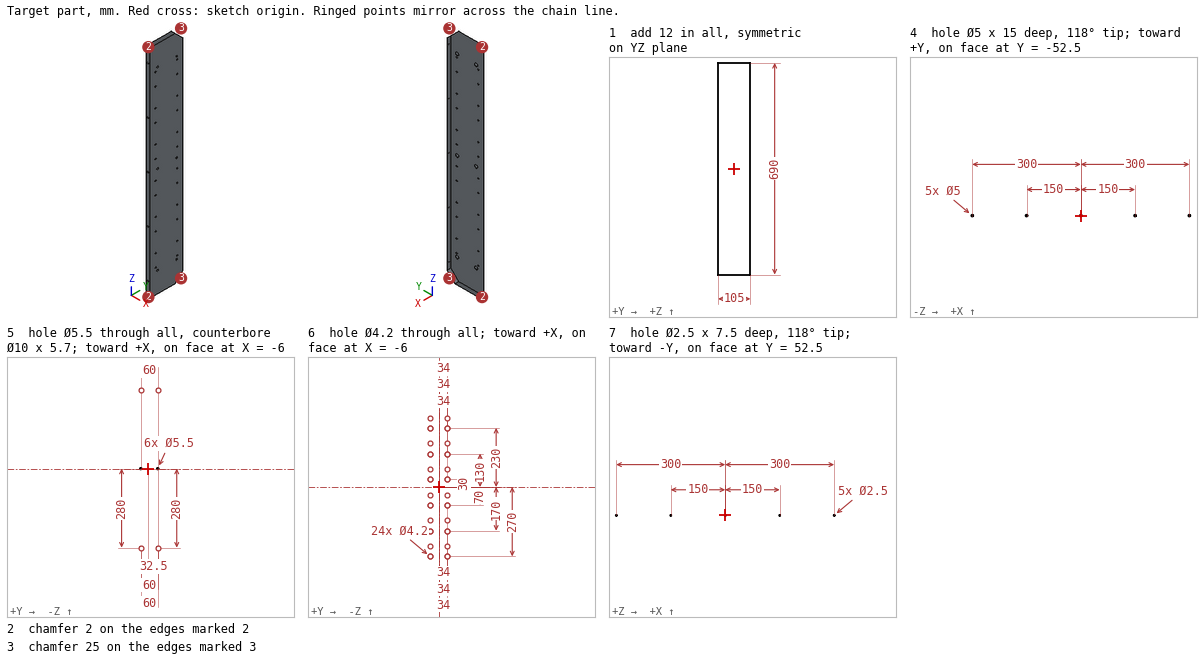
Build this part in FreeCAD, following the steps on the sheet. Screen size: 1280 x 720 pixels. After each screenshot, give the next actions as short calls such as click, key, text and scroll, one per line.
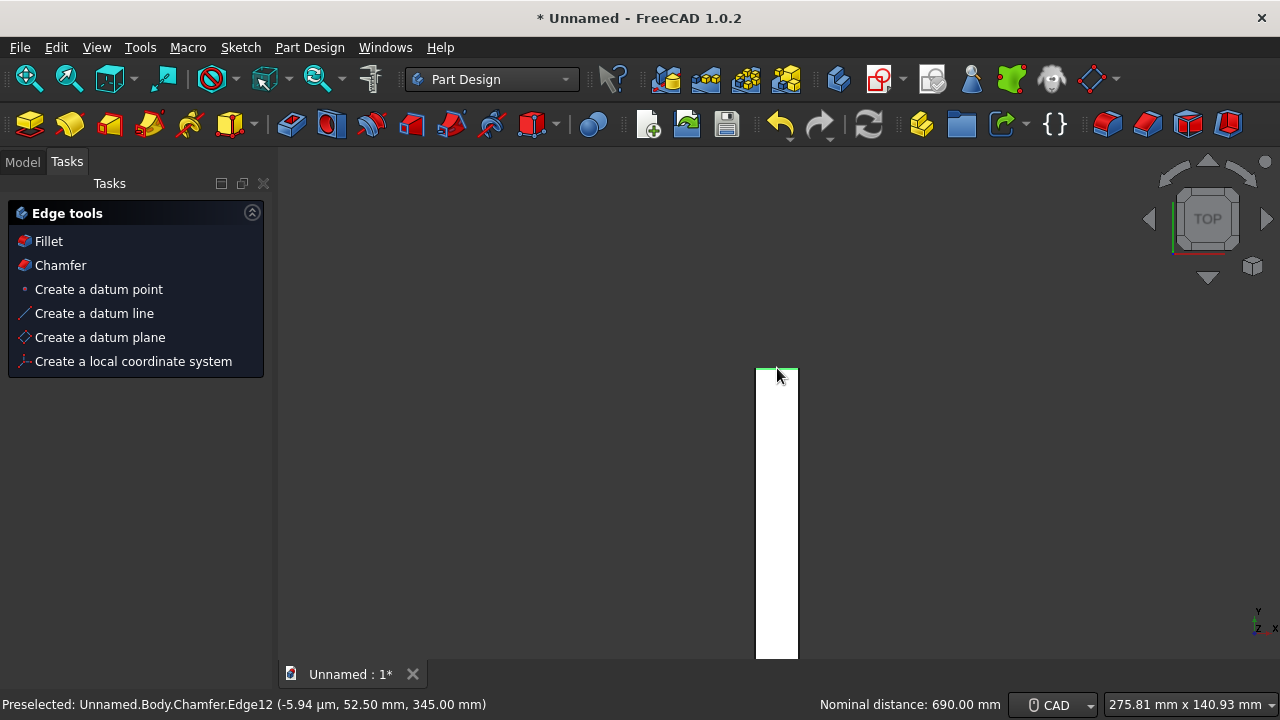
click(1148, 124)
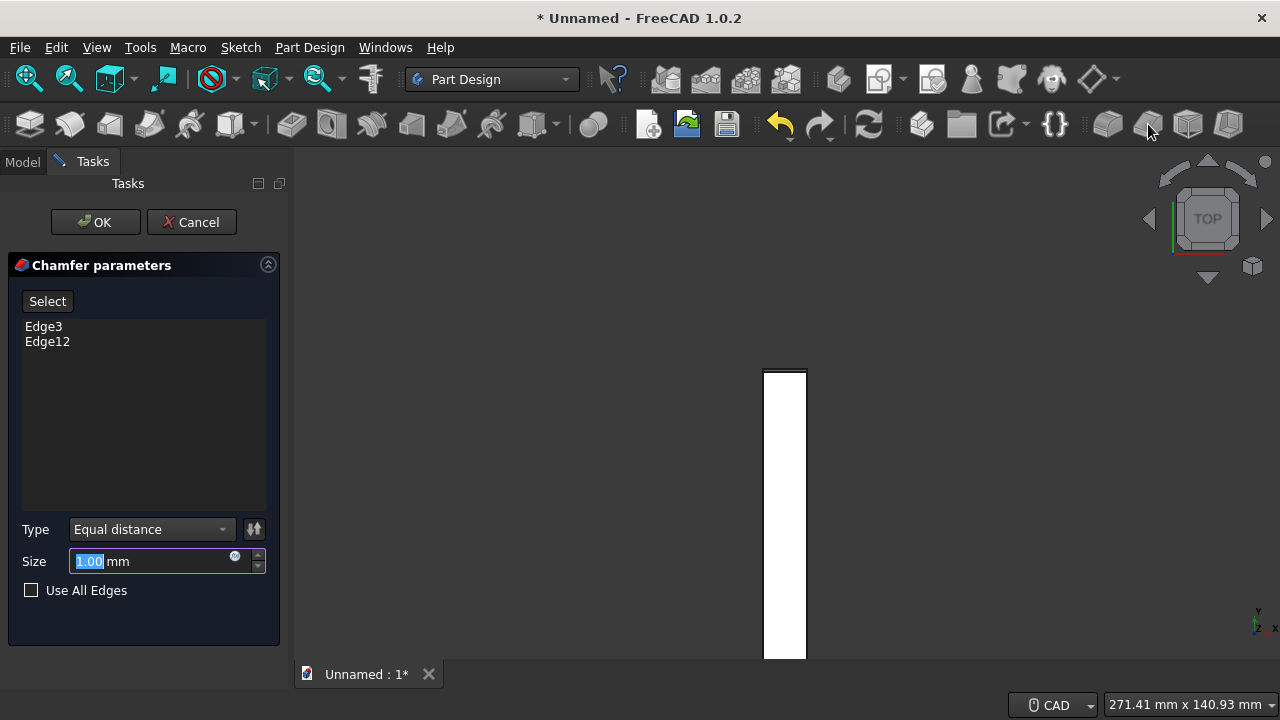
text(25)
key(Tab)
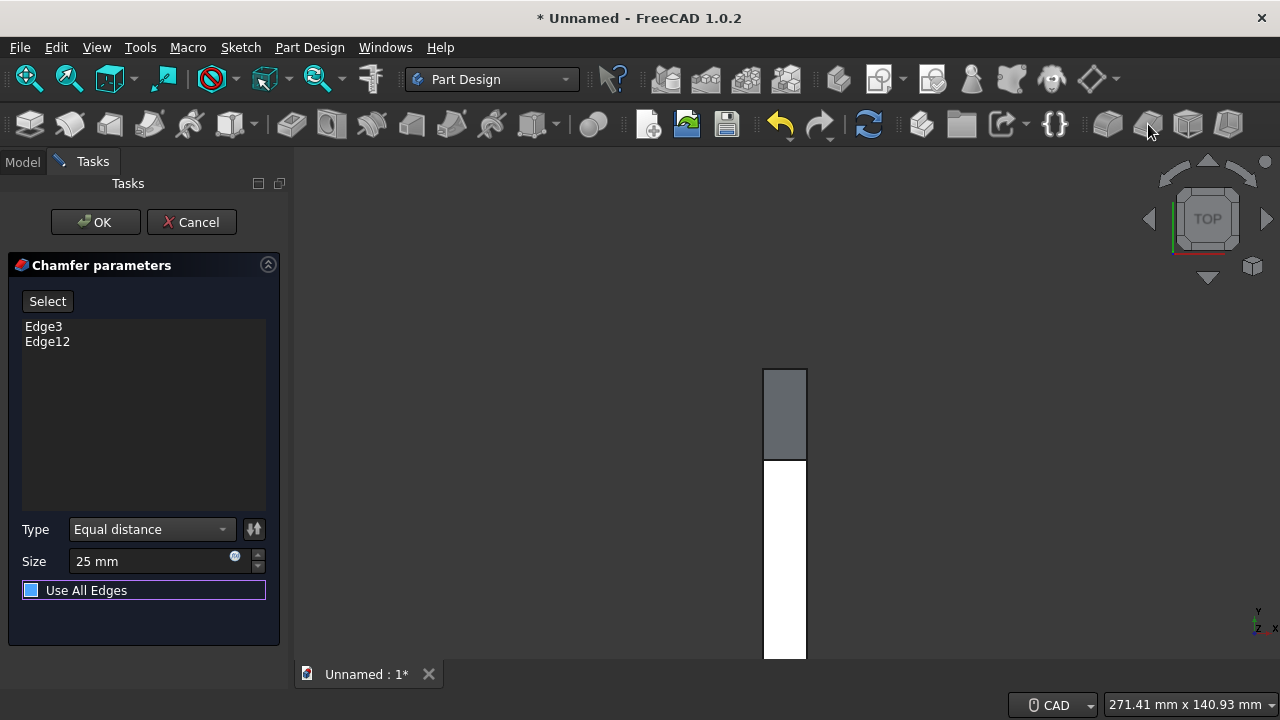
click(96, 222)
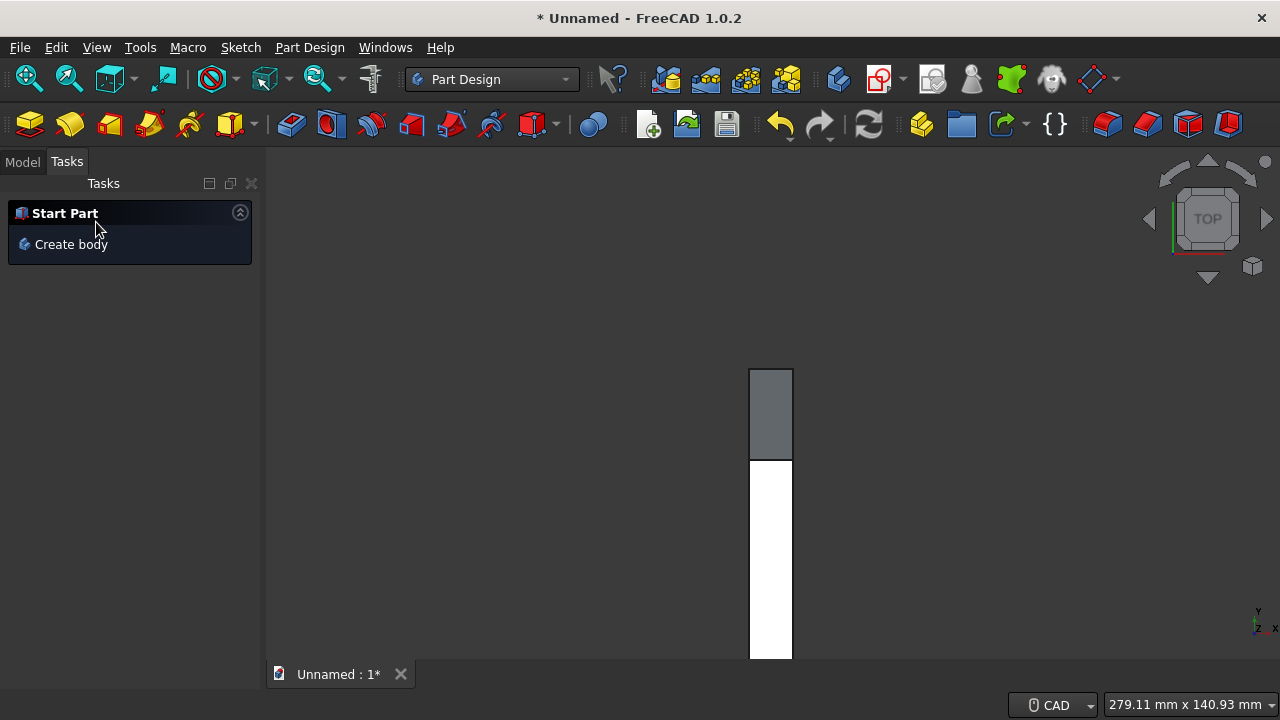
click(30, 80)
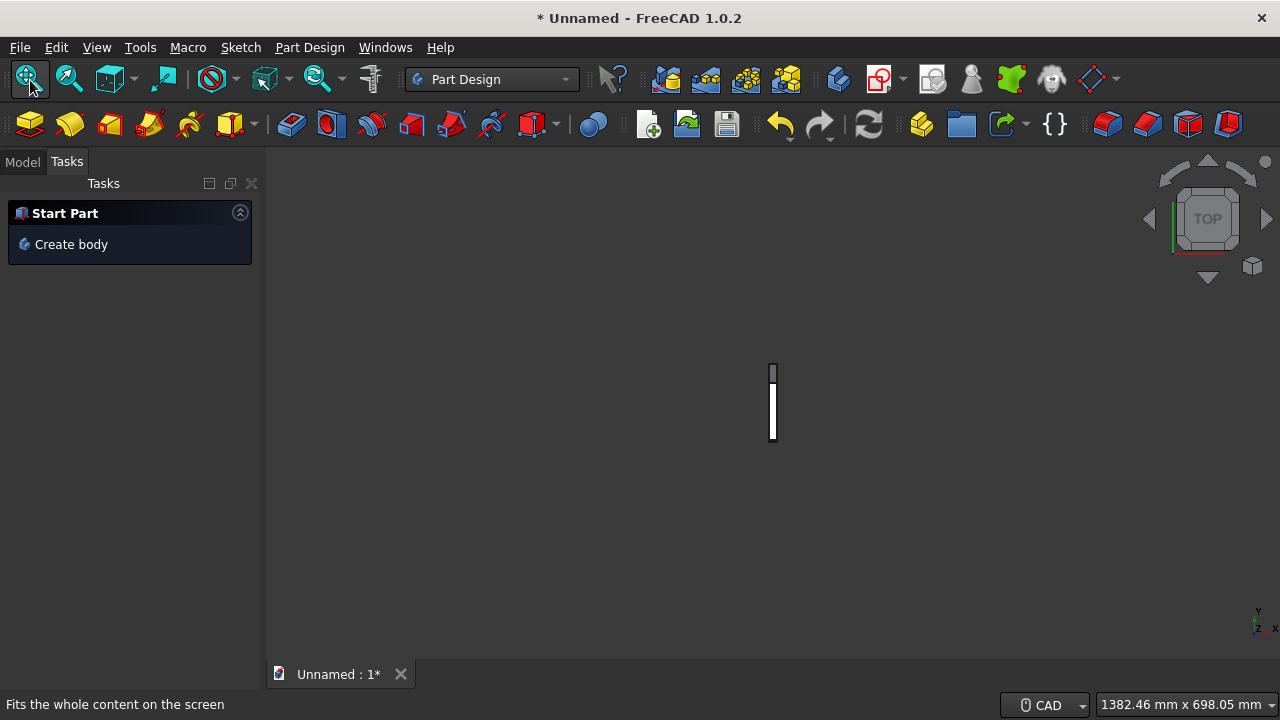
key(0)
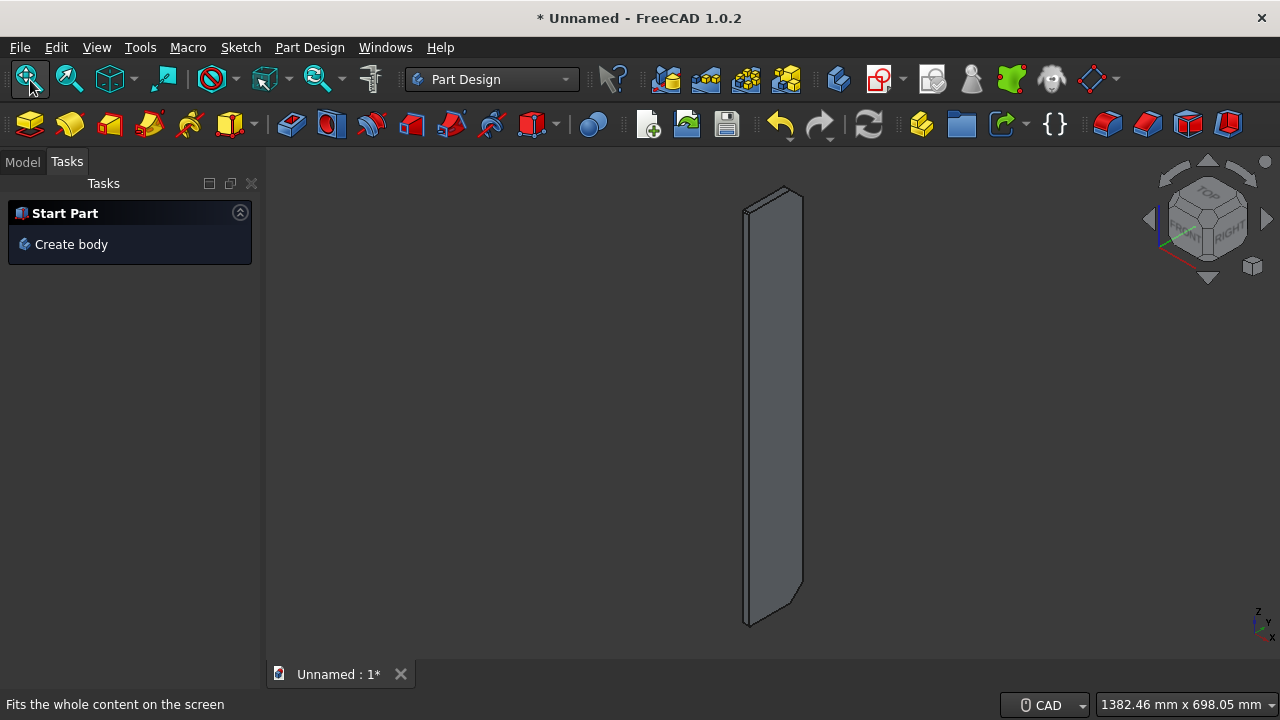
scroll(746, 594, up, 6)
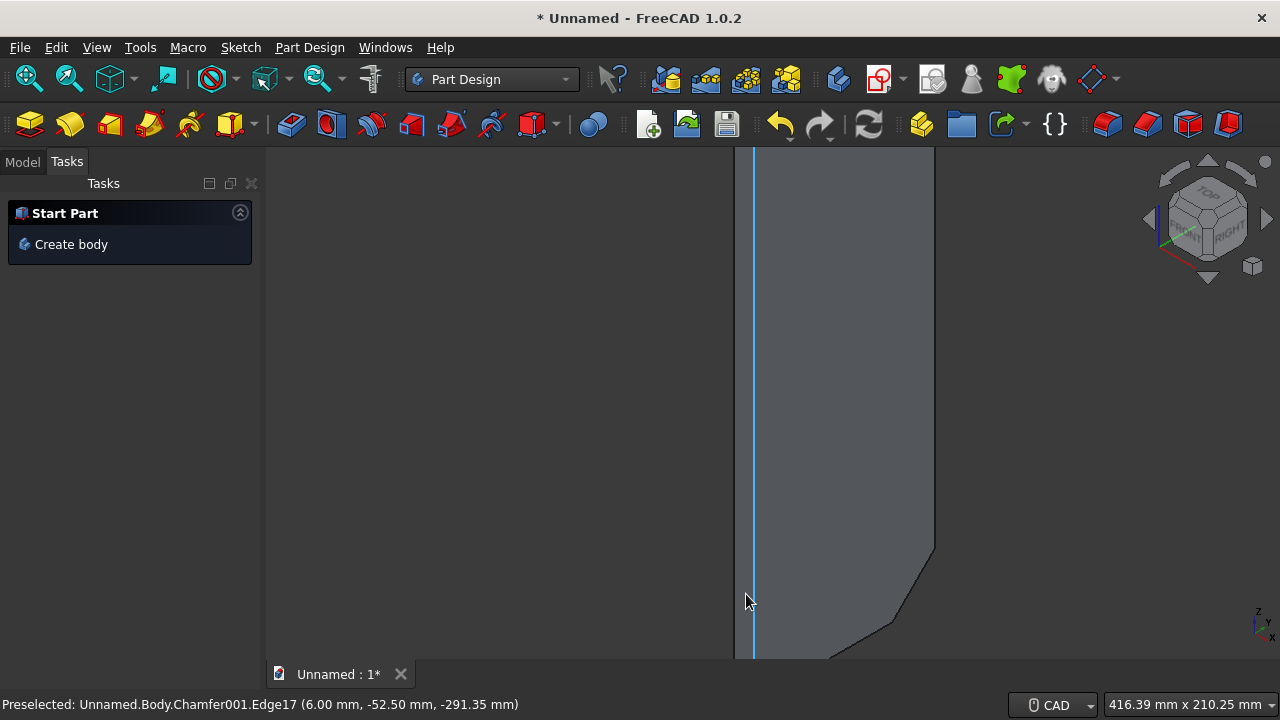
click(744, 594)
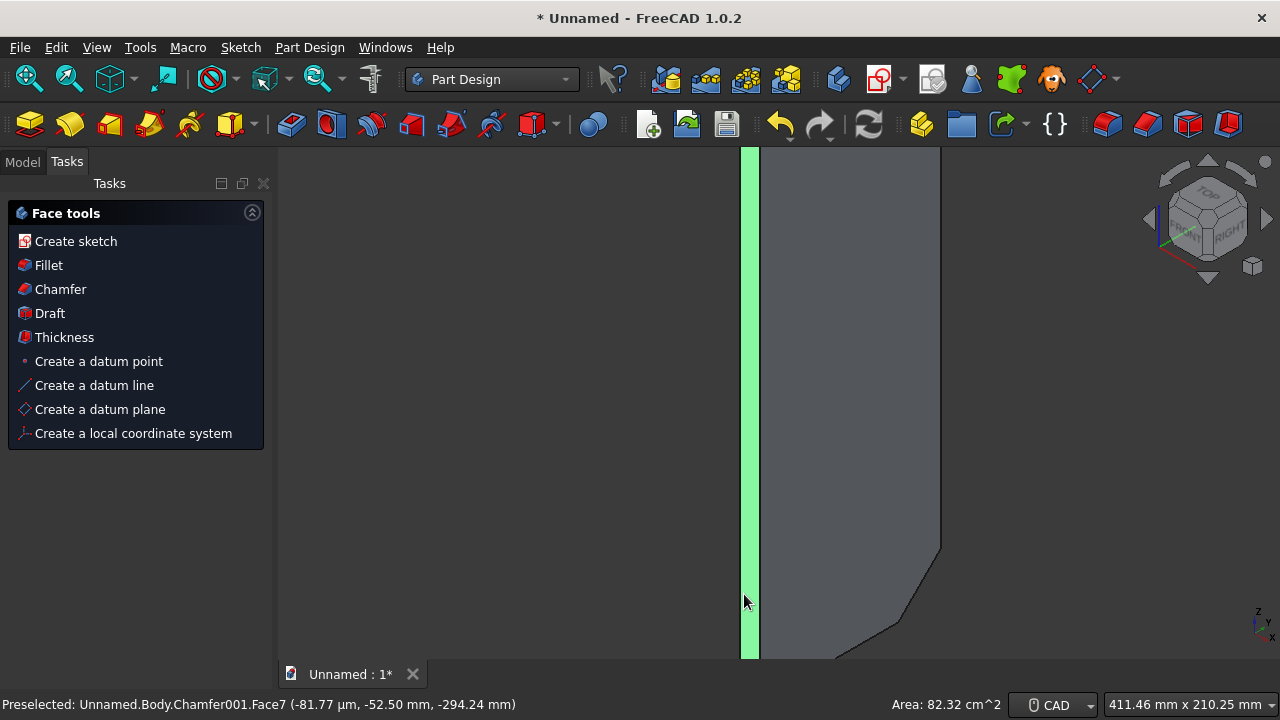
click(880, 80)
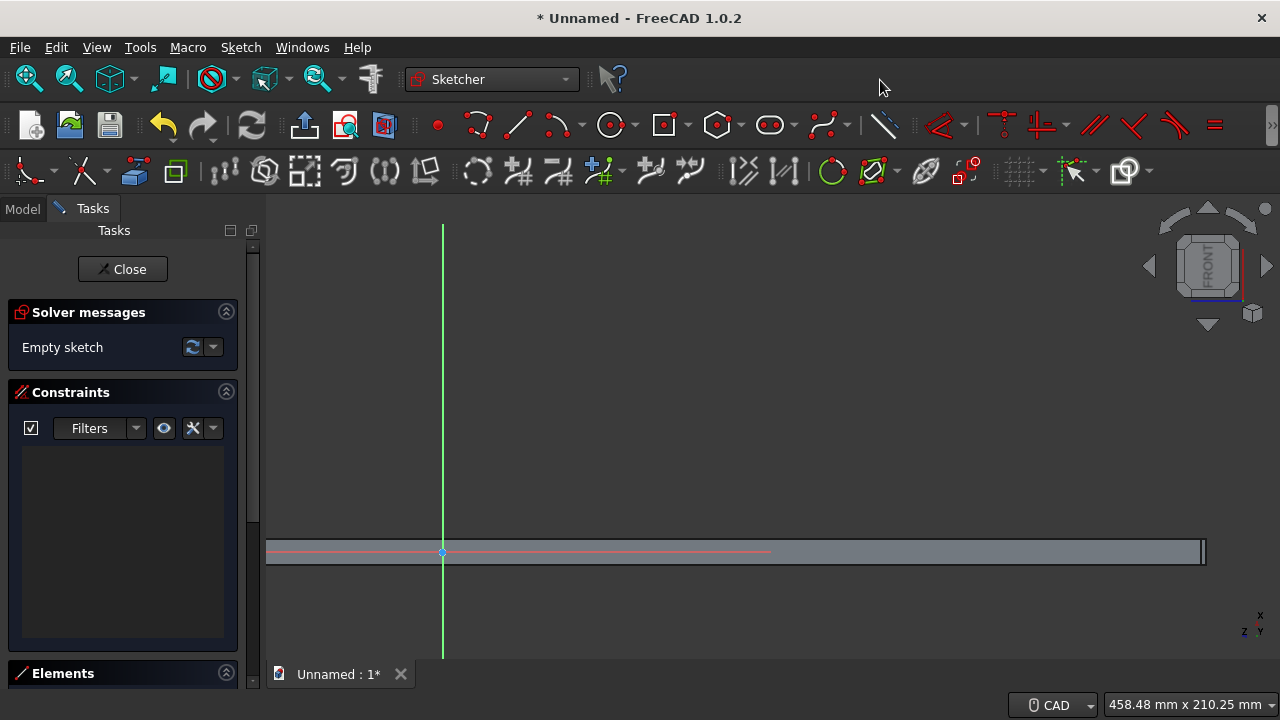
scroll(918, 324, down, 4)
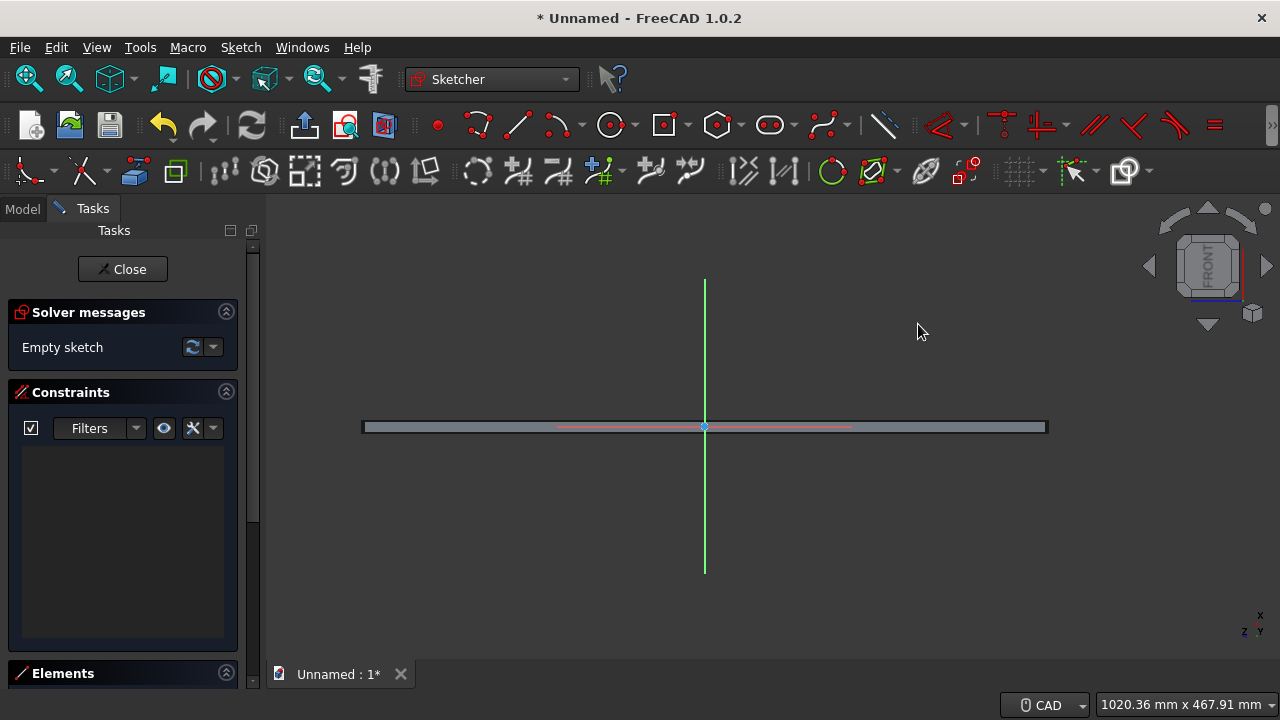
click(612, 126)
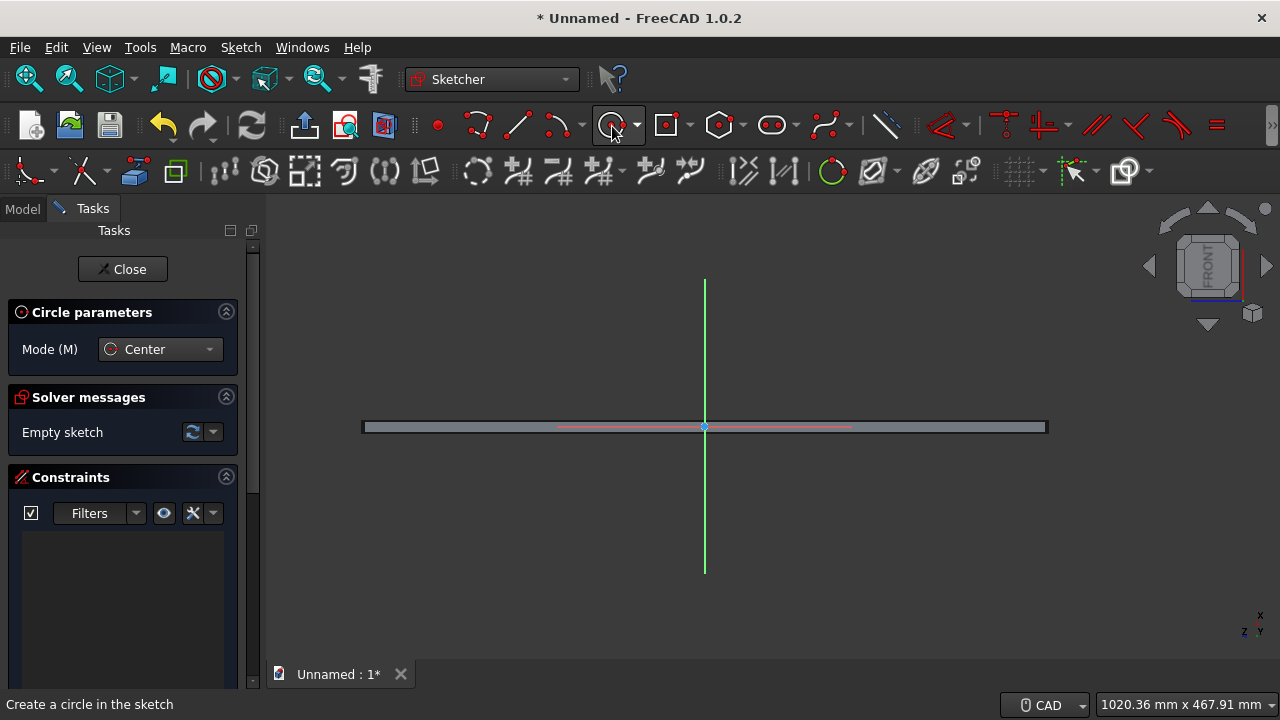
scroll(407, 427, up, 12)